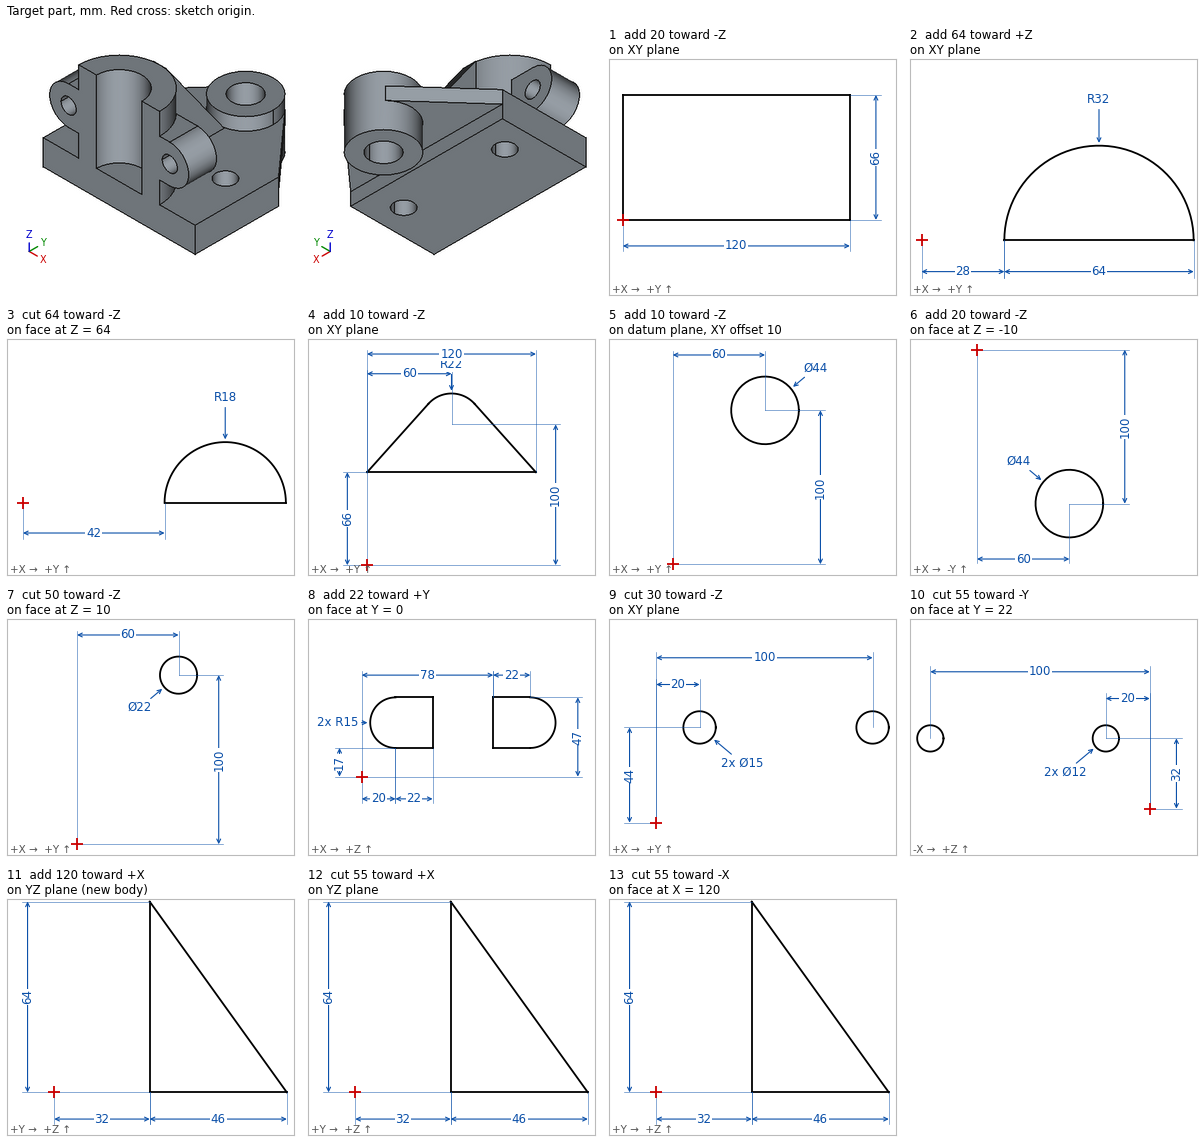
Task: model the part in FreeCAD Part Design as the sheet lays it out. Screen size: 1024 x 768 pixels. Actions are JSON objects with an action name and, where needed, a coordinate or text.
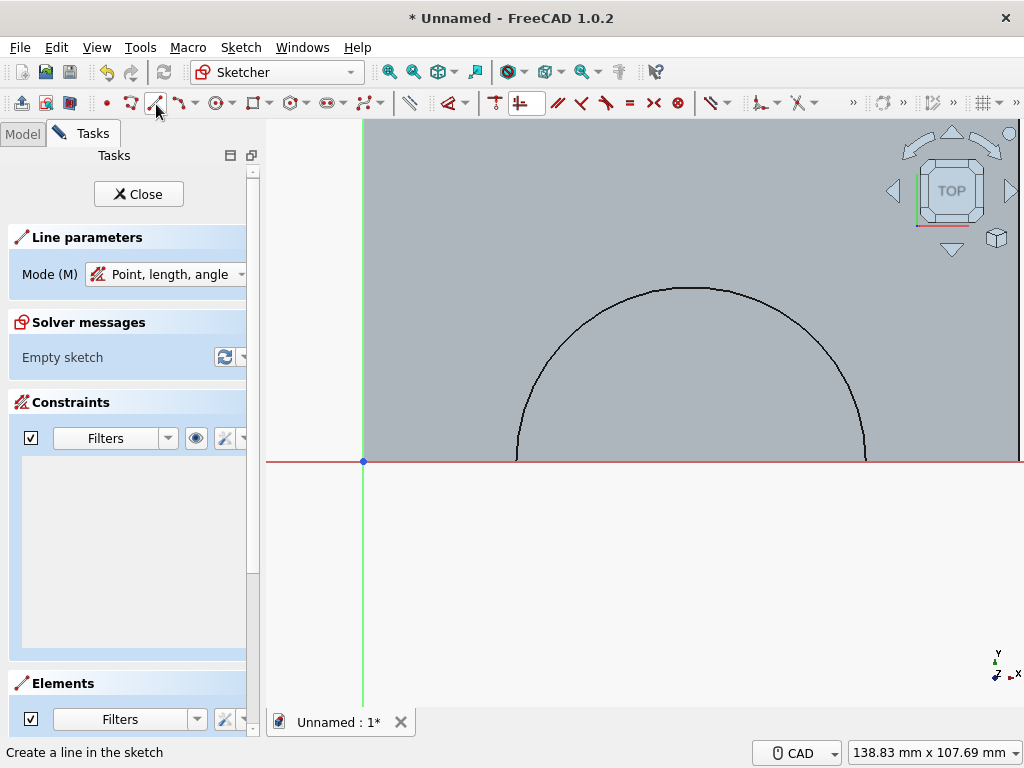
{"action": "left_click", "coordinate": [593, 462]}
{"action": "left_click", "coordinate": [789, 453]}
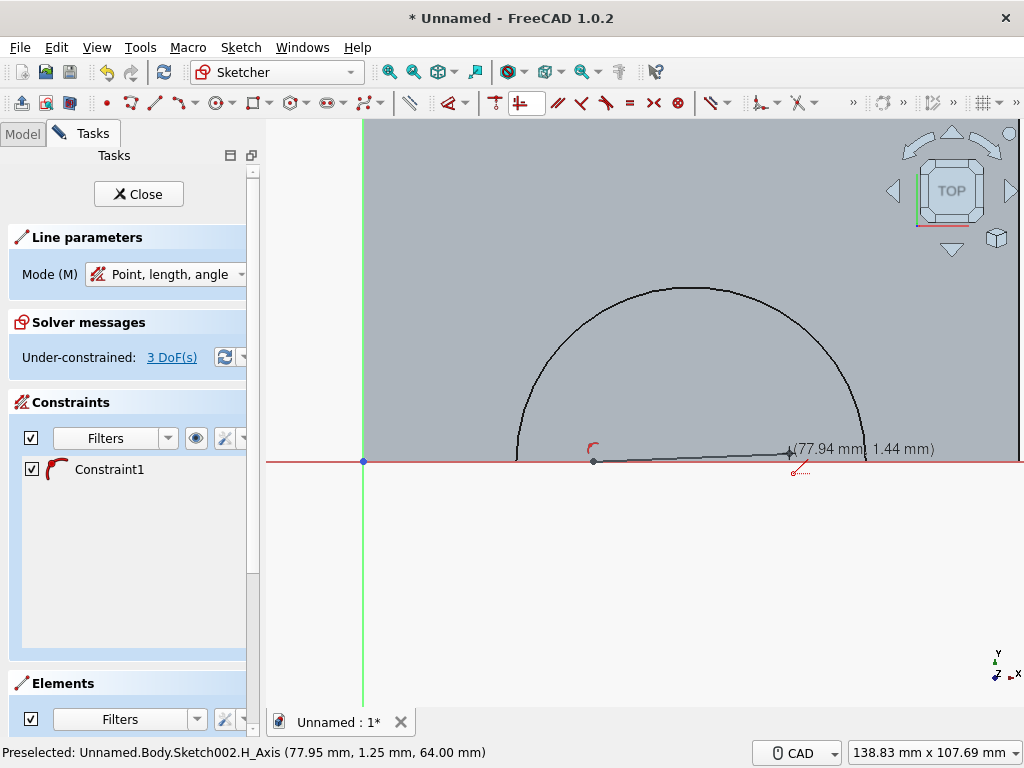
{"action": "left_click", "coordinate": [180, 104]}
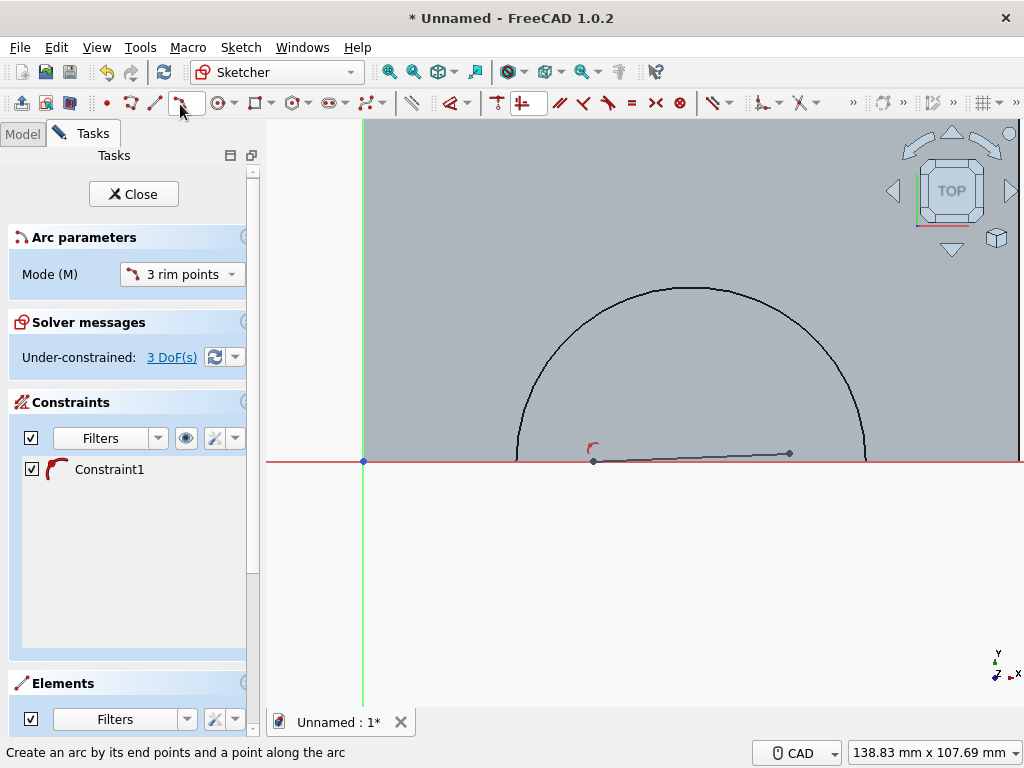
{"action": "left_click", "coordinate": [789, 454]}
{"action": "left_click", "coordinate": [593, 462]}
{"action": "left_click", "coordinate": [691, 364]}
{"action": "key", "text": "Escape"}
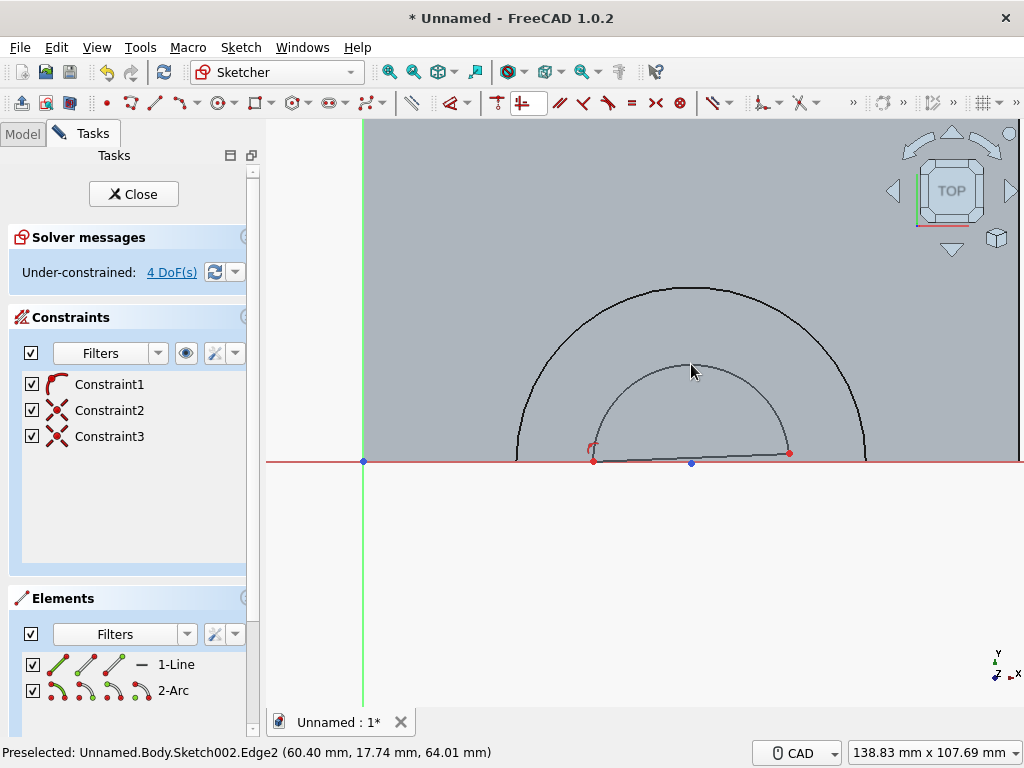
{"action": "left_click", "coordinate": [652, 460]}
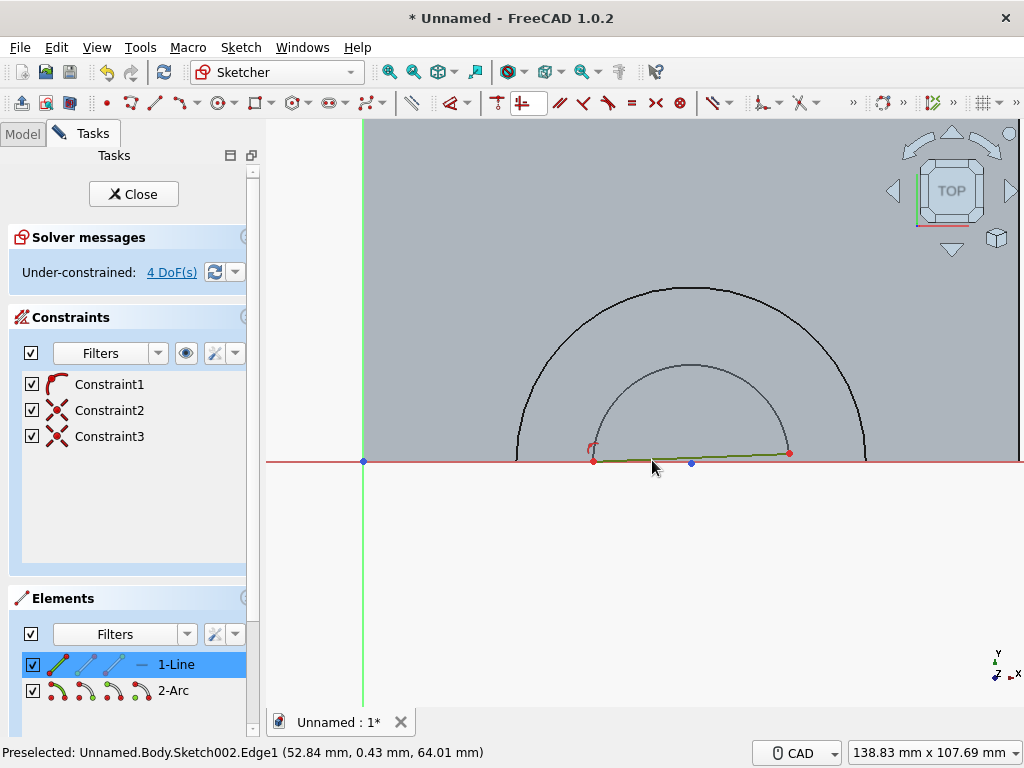
{"action": "left_click", "coordinate": [542, 104]}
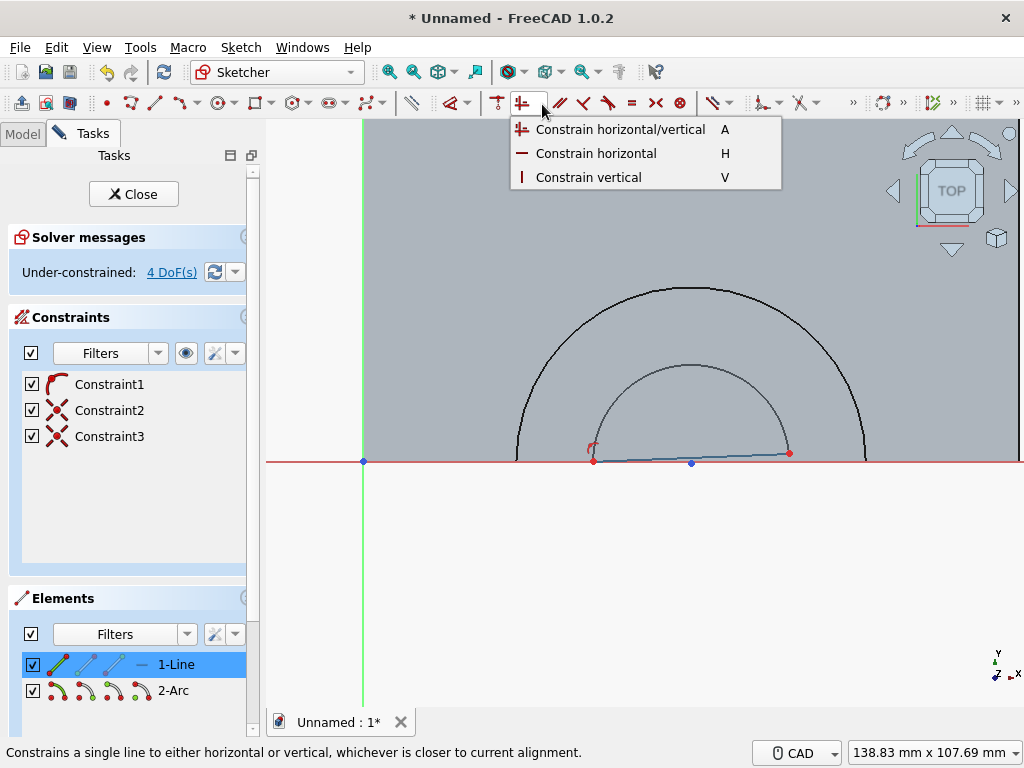
{"action": "left_click", "coordinate": [646, 153]}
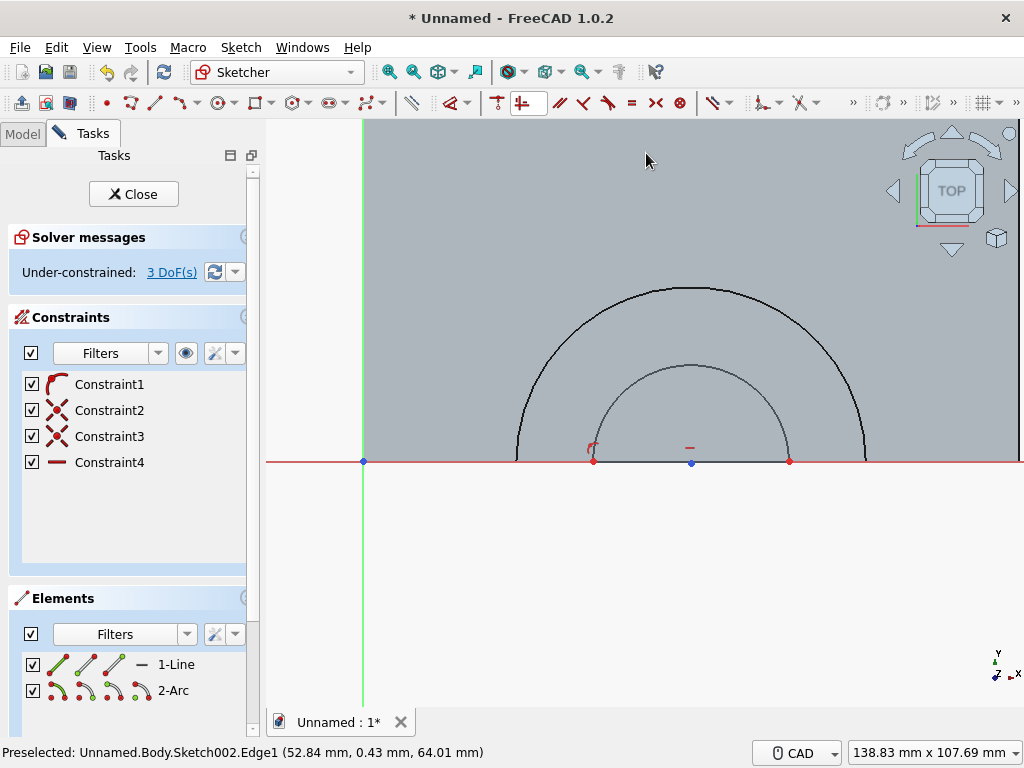
{"action": "left_click", "coordinate": [691, 463]}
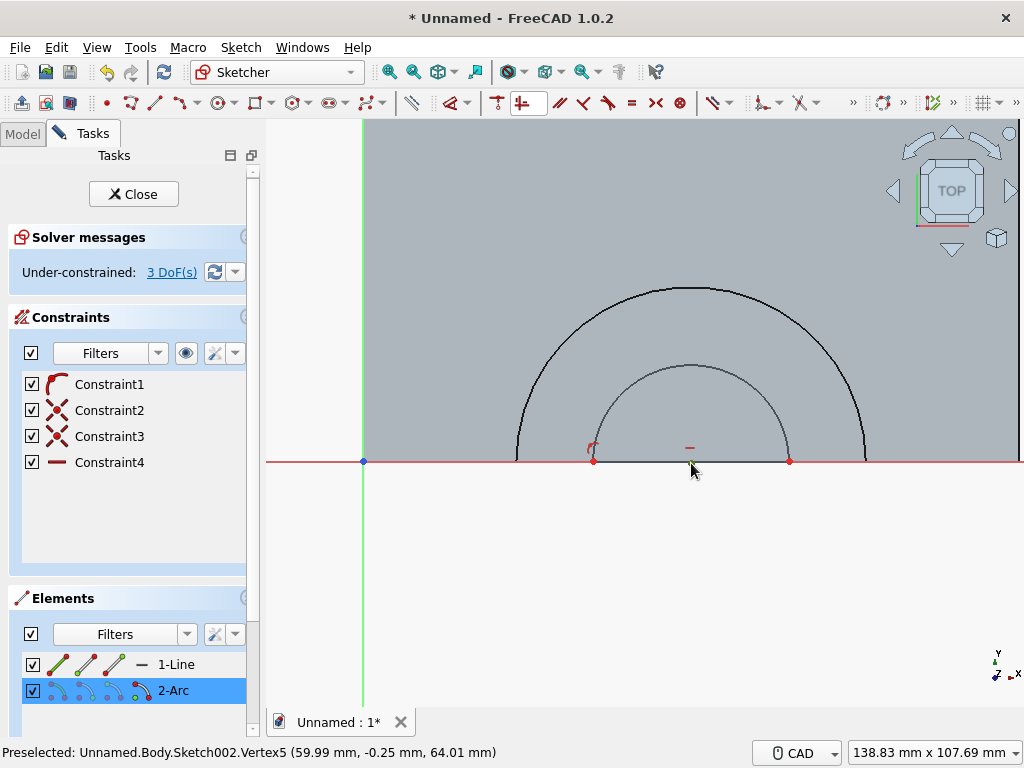
{"action": "left_click", "coordinate": [415, 462]}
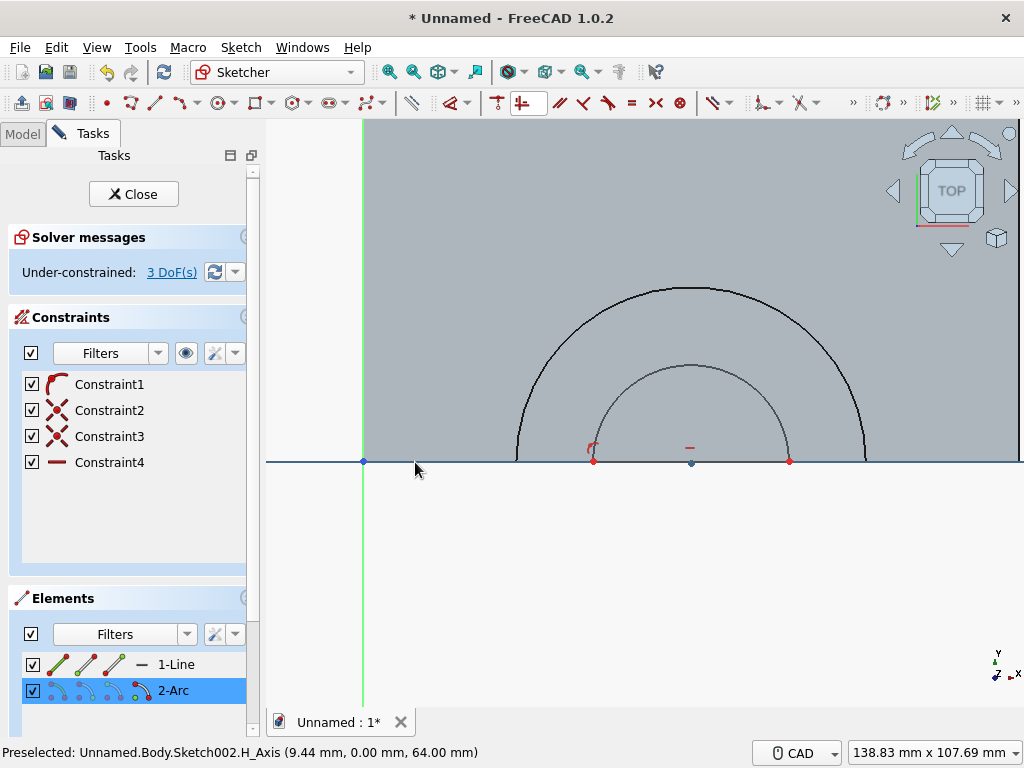
{"action": "left_click", "coordinate": [498, 104]}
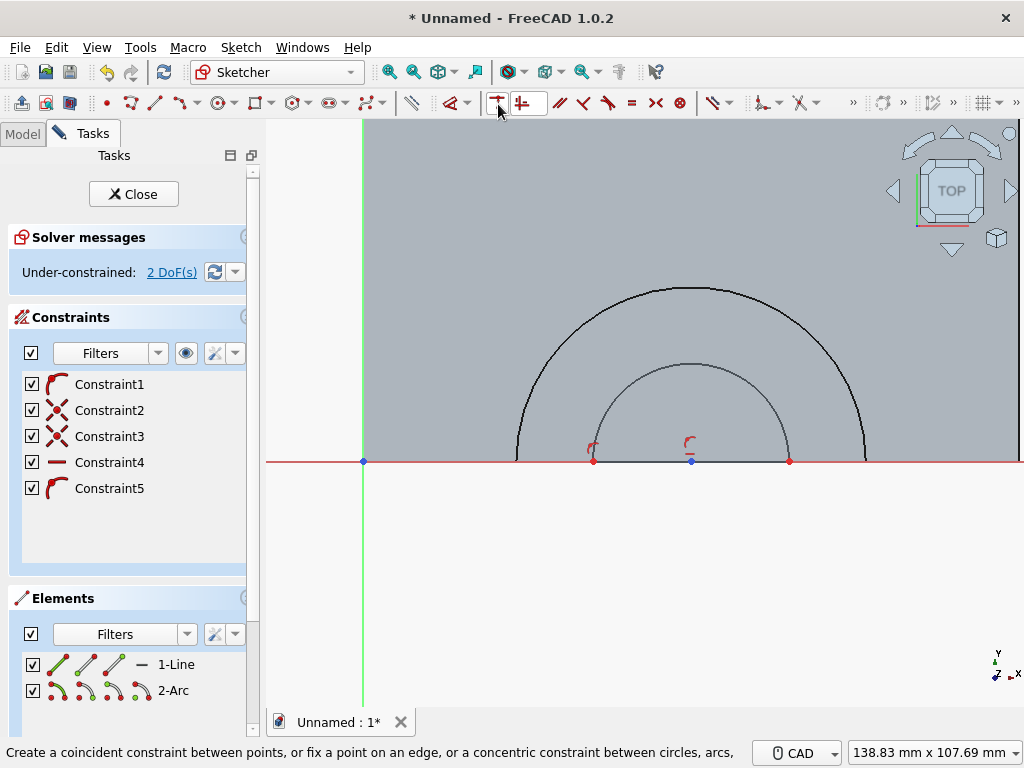
{"action": "left_click", "coordinate": [450, 104]}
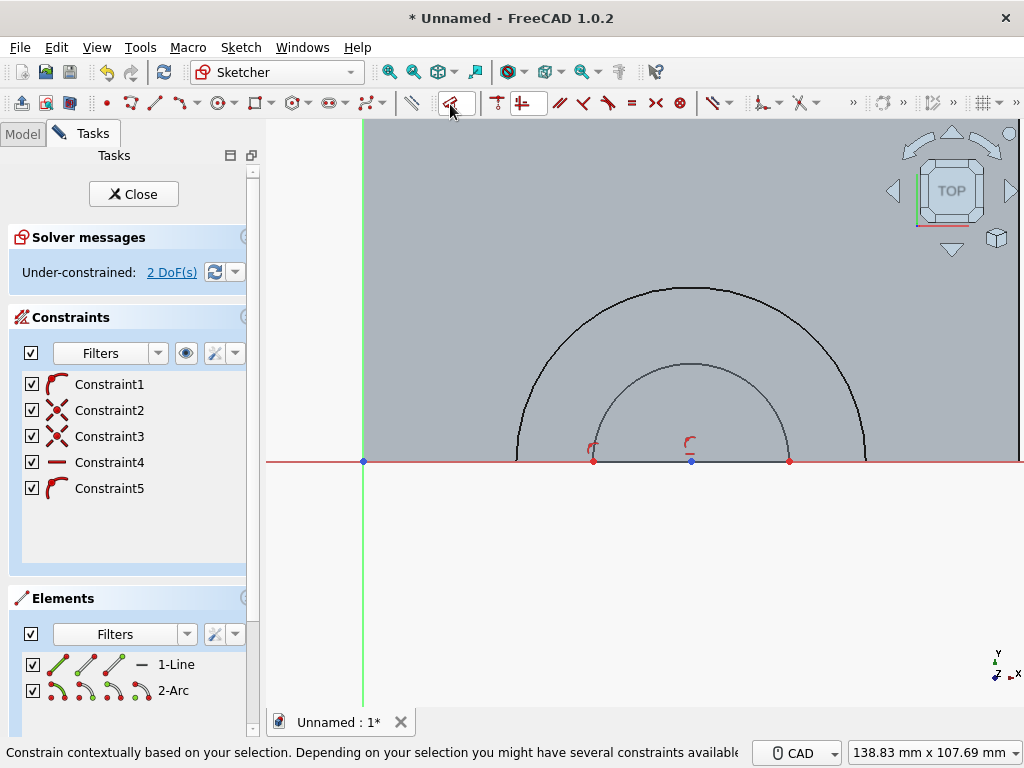
{"action": "left_click", "coordinate": [749, 383]}
{"action": "left_click", "coordinate": [768, 357]}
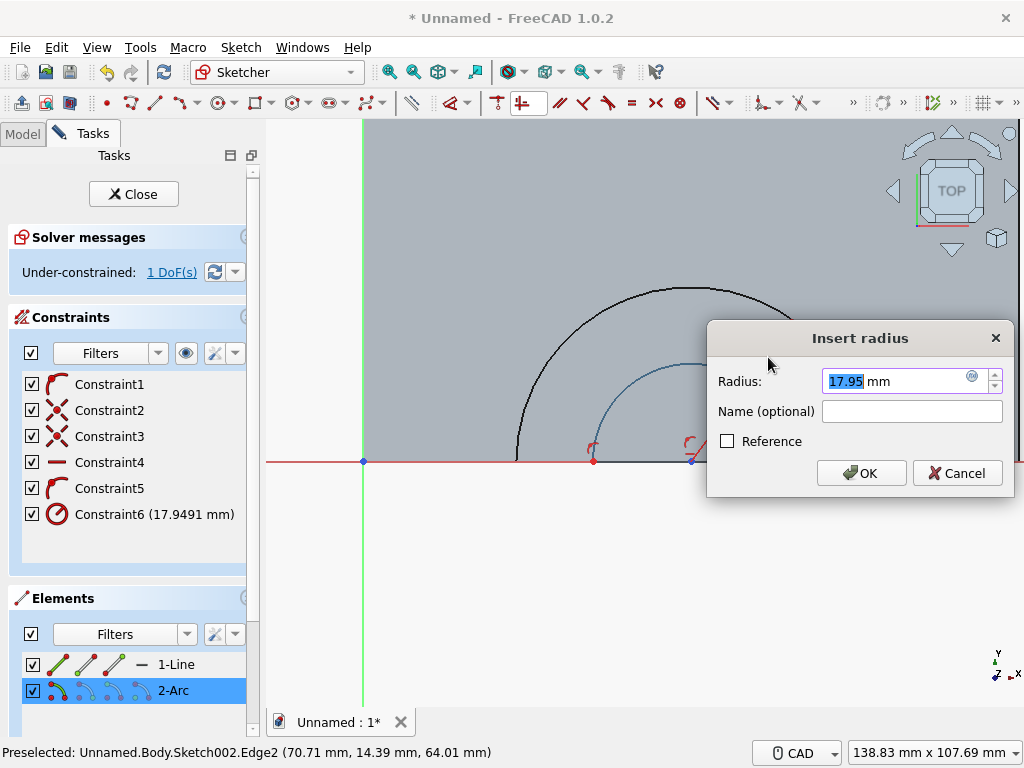
{"action": "type", "text": "18"}
{"action": "key", "text": "Return"}